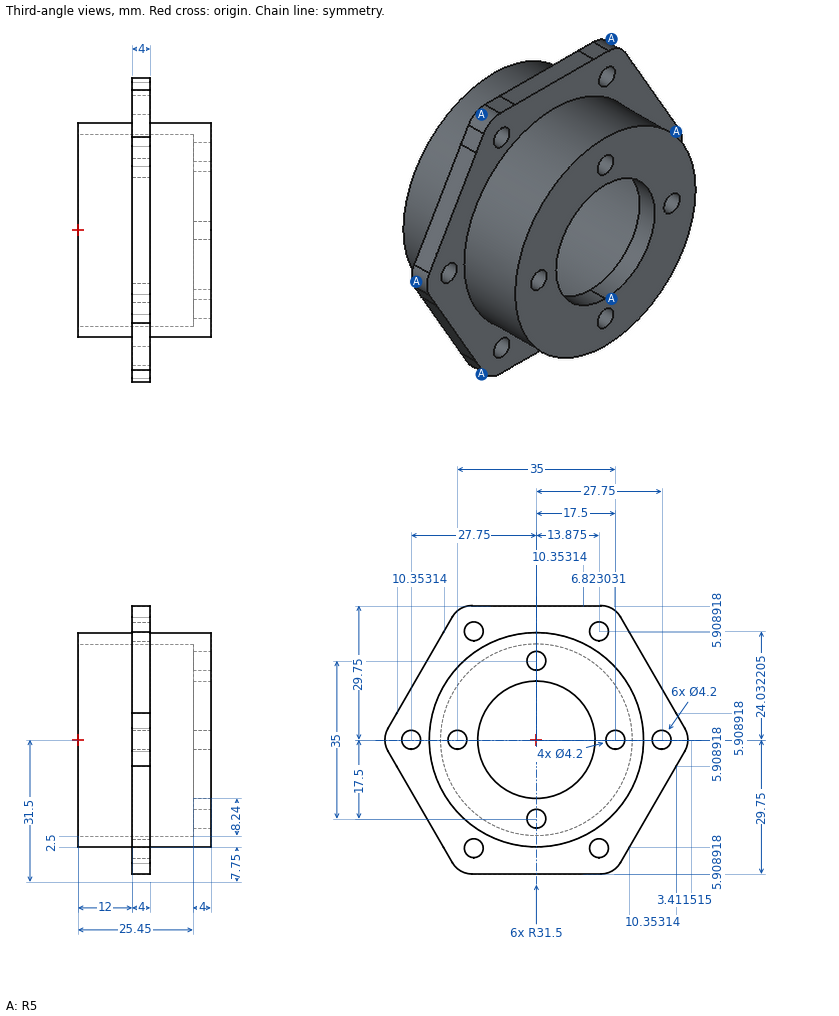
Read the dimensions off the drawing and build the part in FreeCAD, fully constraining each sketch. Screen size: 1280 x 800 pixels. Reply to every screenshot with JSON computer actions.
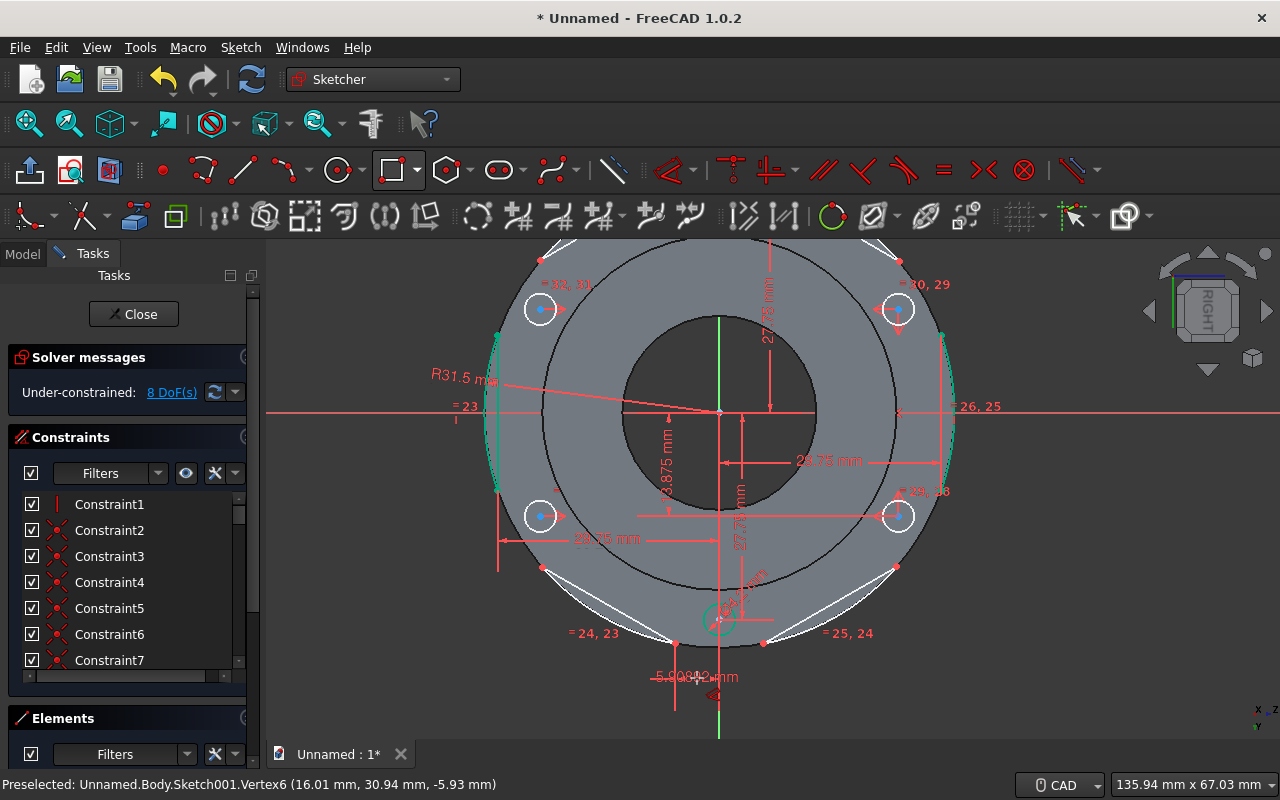
{"action": "left_click", "coordinate": [764, 644]}
{"action": "left_click", "coordinate": [742, 379]}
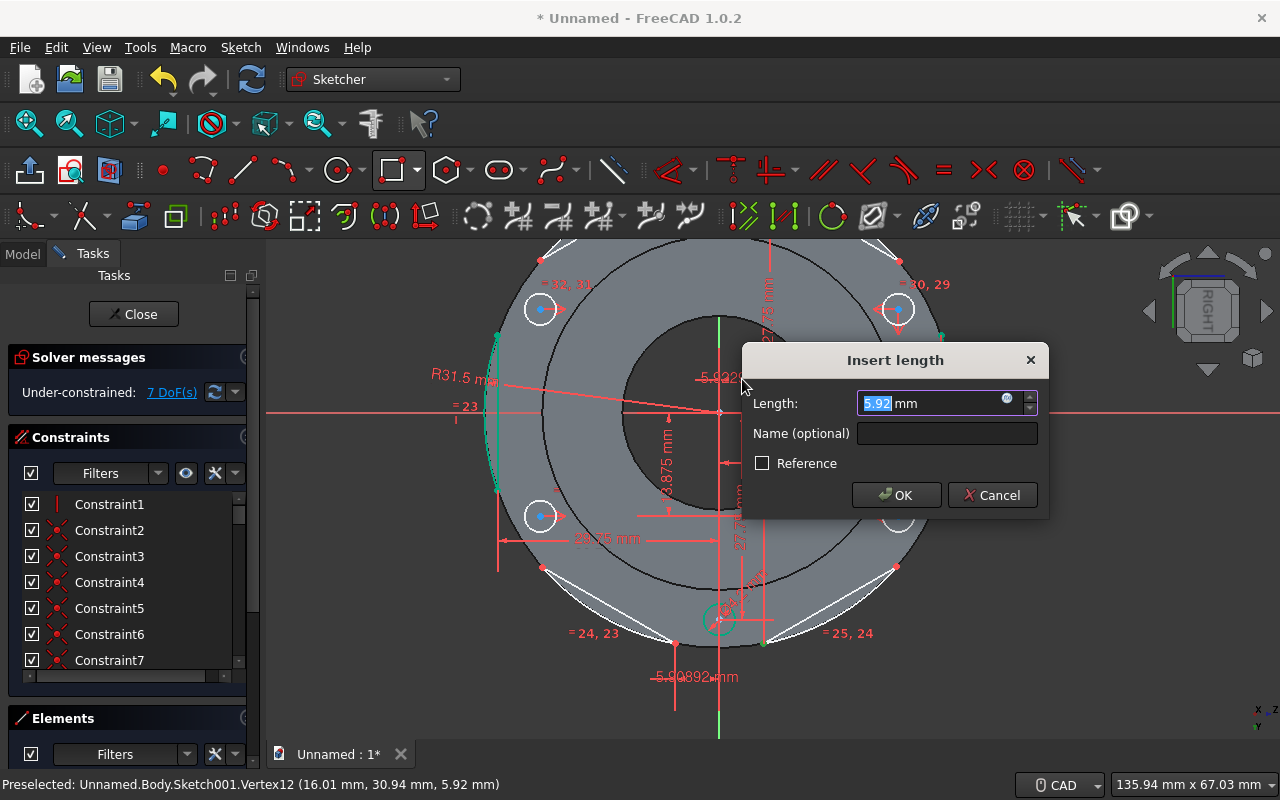
{"action": "type", "text": "5.908918"}
{"action": "key", "text": "Return"}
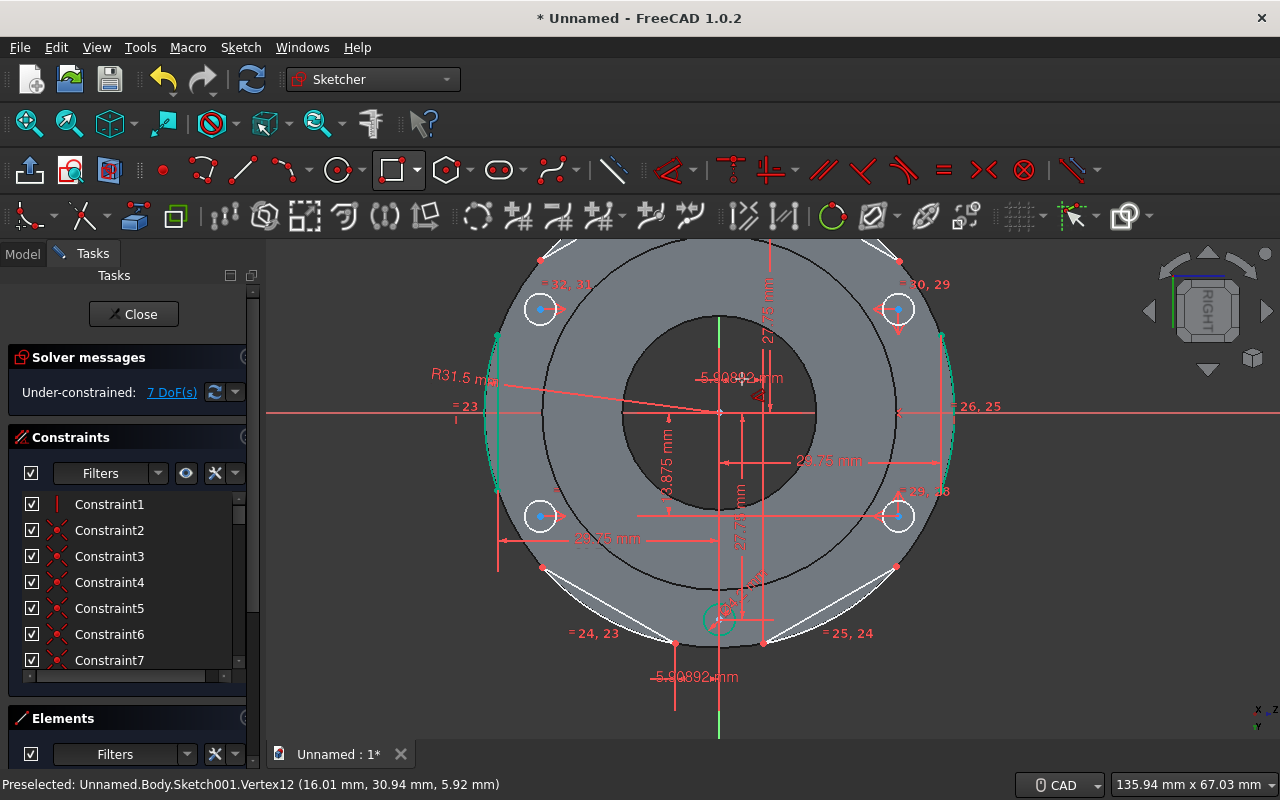
{"action": "scroll", "coordinate": [674, 644], "scroll_direction": "down", "scroll_amount": 2}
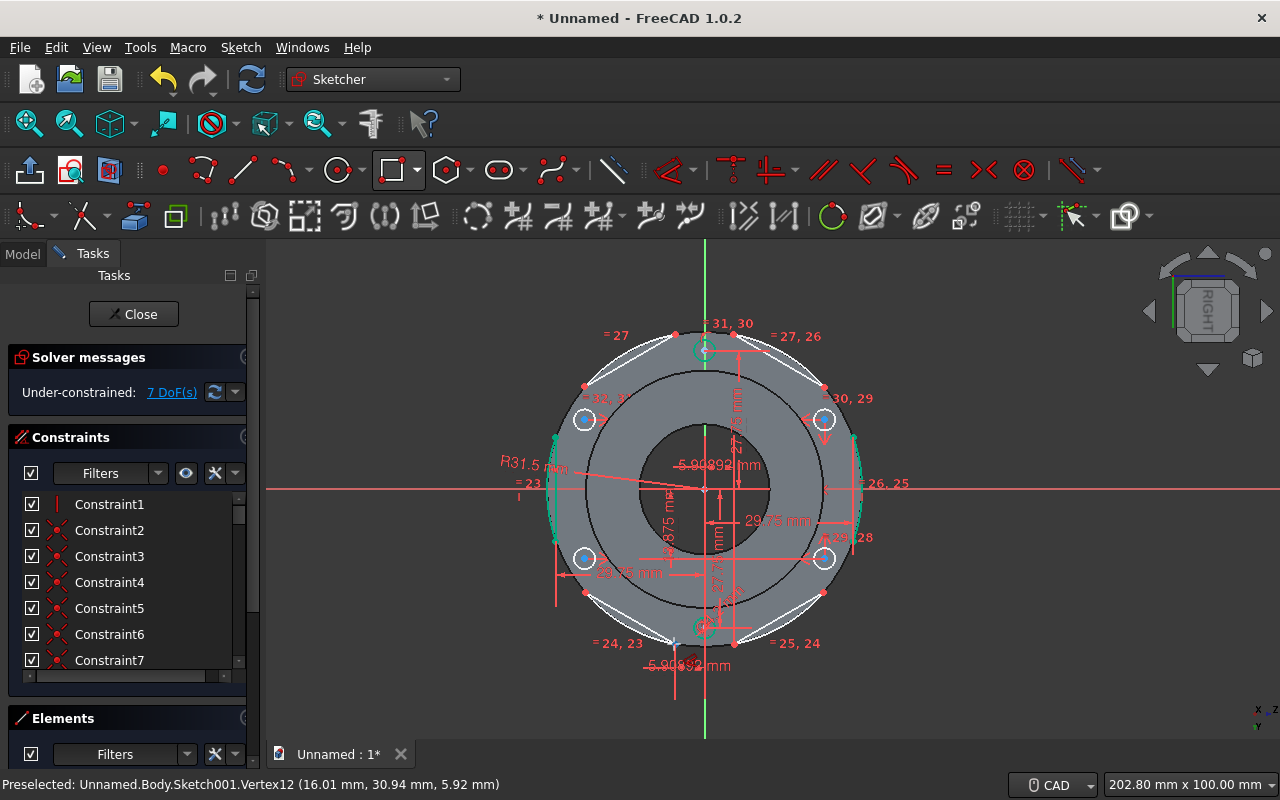
{"action": "scroll", "coordinate": [734, 335], "scroll_direction": "up", "scroll_amount": 2}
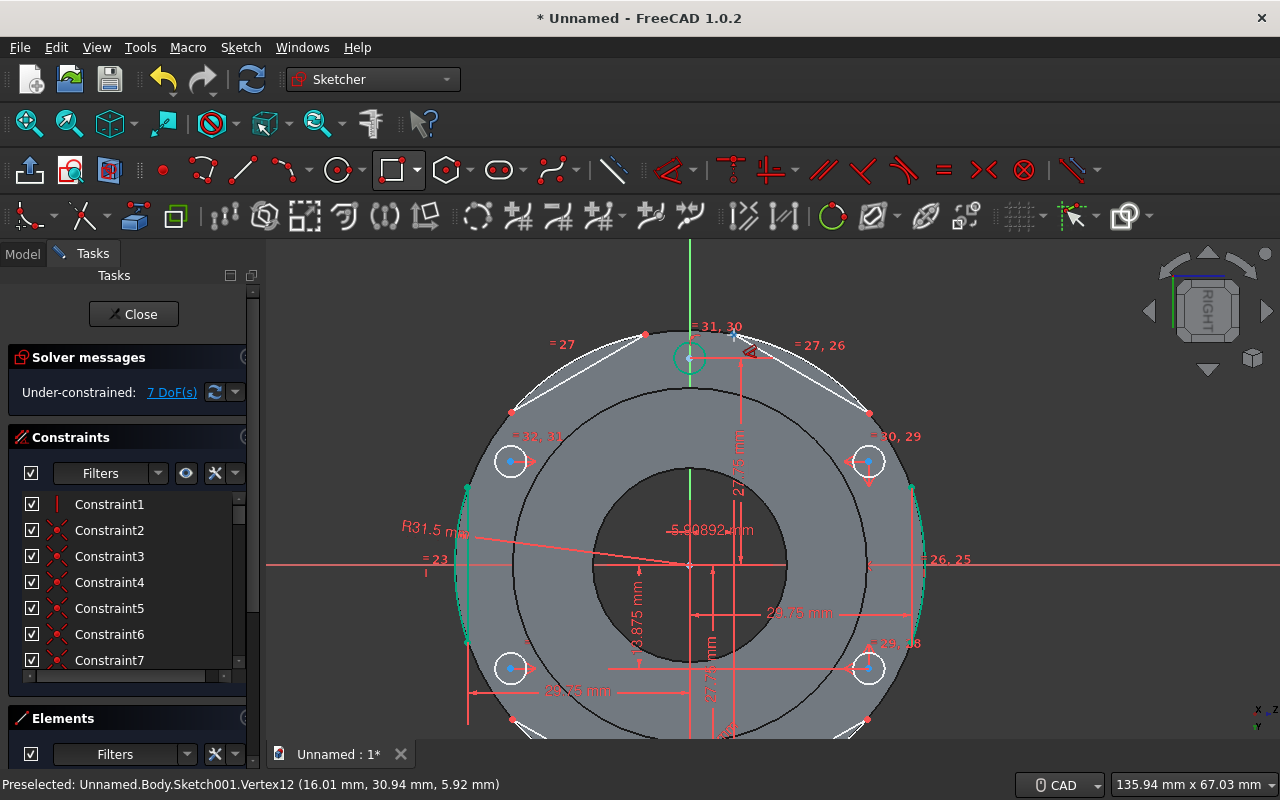
{"action": "left_click", "coordinate": [734, 334]}
{"action": "left_click", "coordinate": [712, 300]}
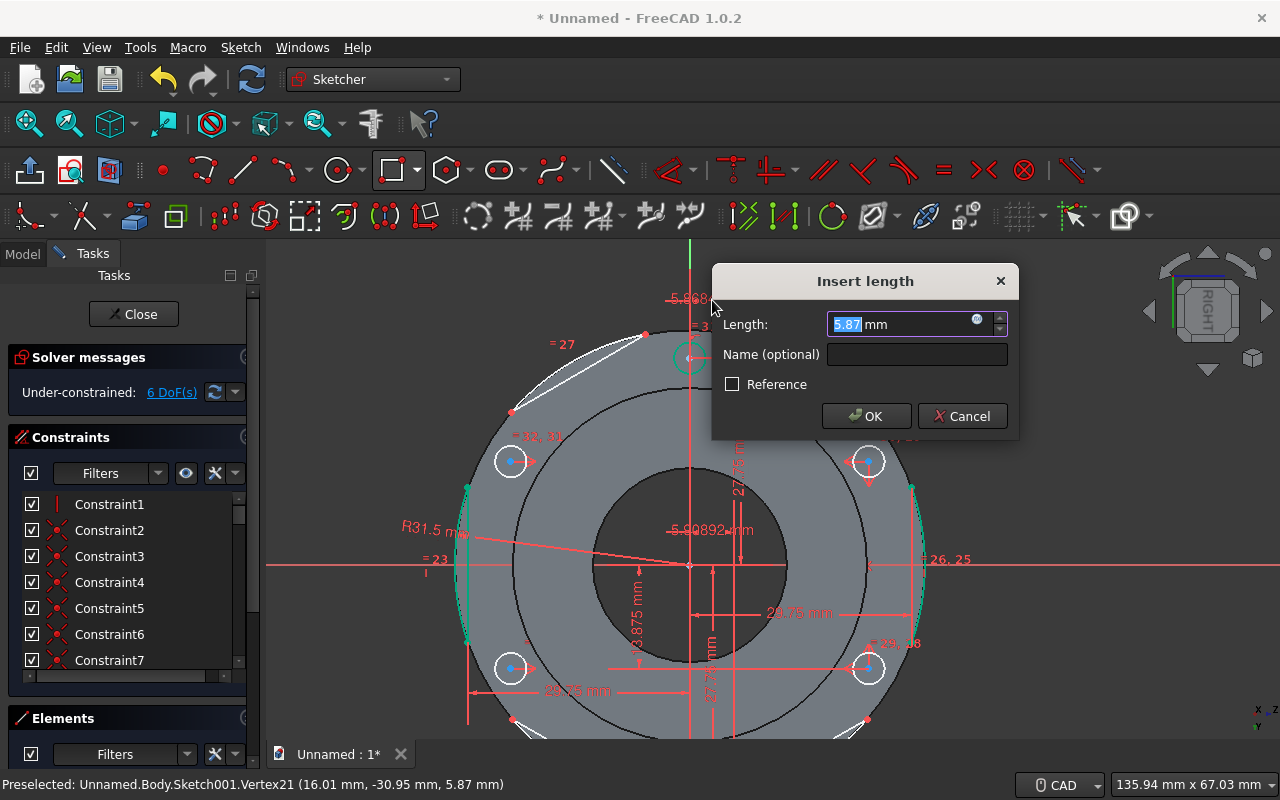
{"action": "type", "text": "5.908918"}
{"action": "key", "text": "Return"}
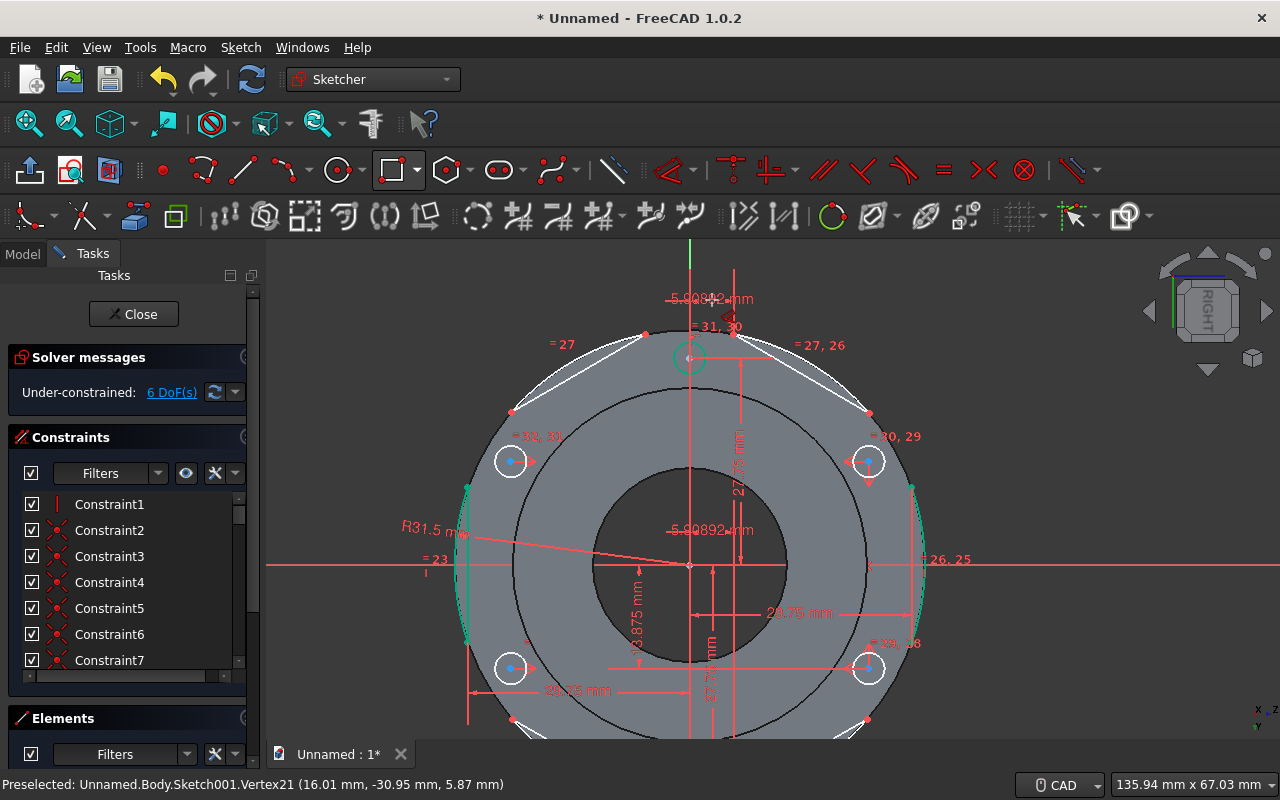
{"action": "left_click", "coordinate": [646, 334]}
{"action": "left_click", "coordinate": [668, 276]}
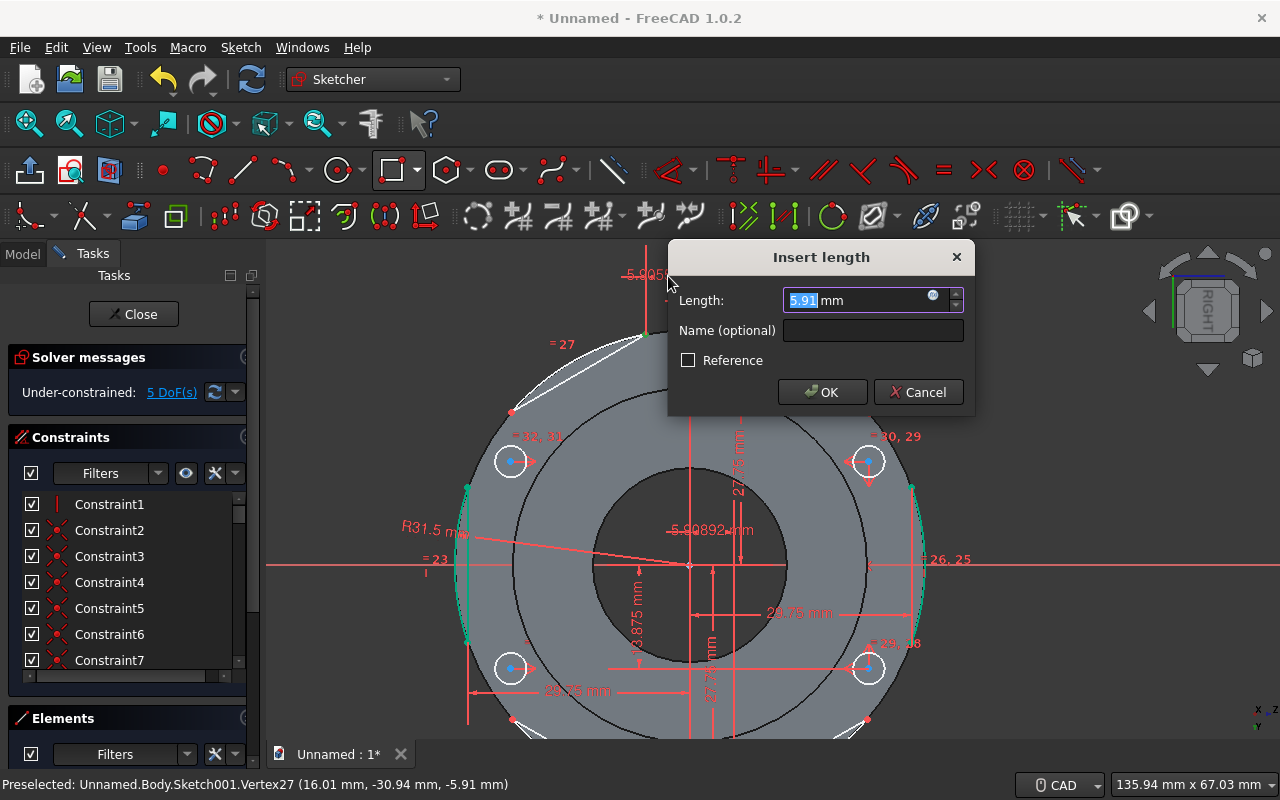
{"action": "type", "text": "5.908918"}
{"action": "key", "text": "Return"}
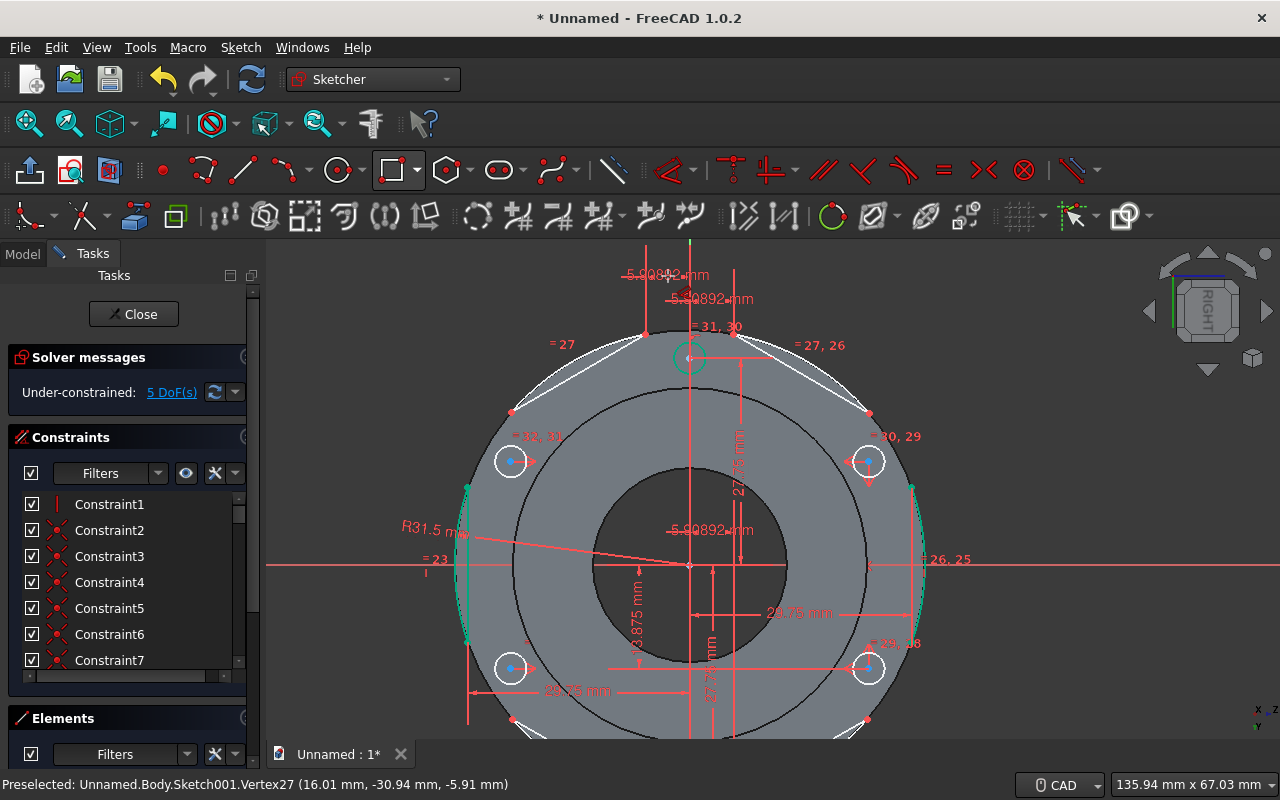
{"action": "scroll", "coordinate": [734, 334], "scroll_direction": "down", "scroll_amount": 2}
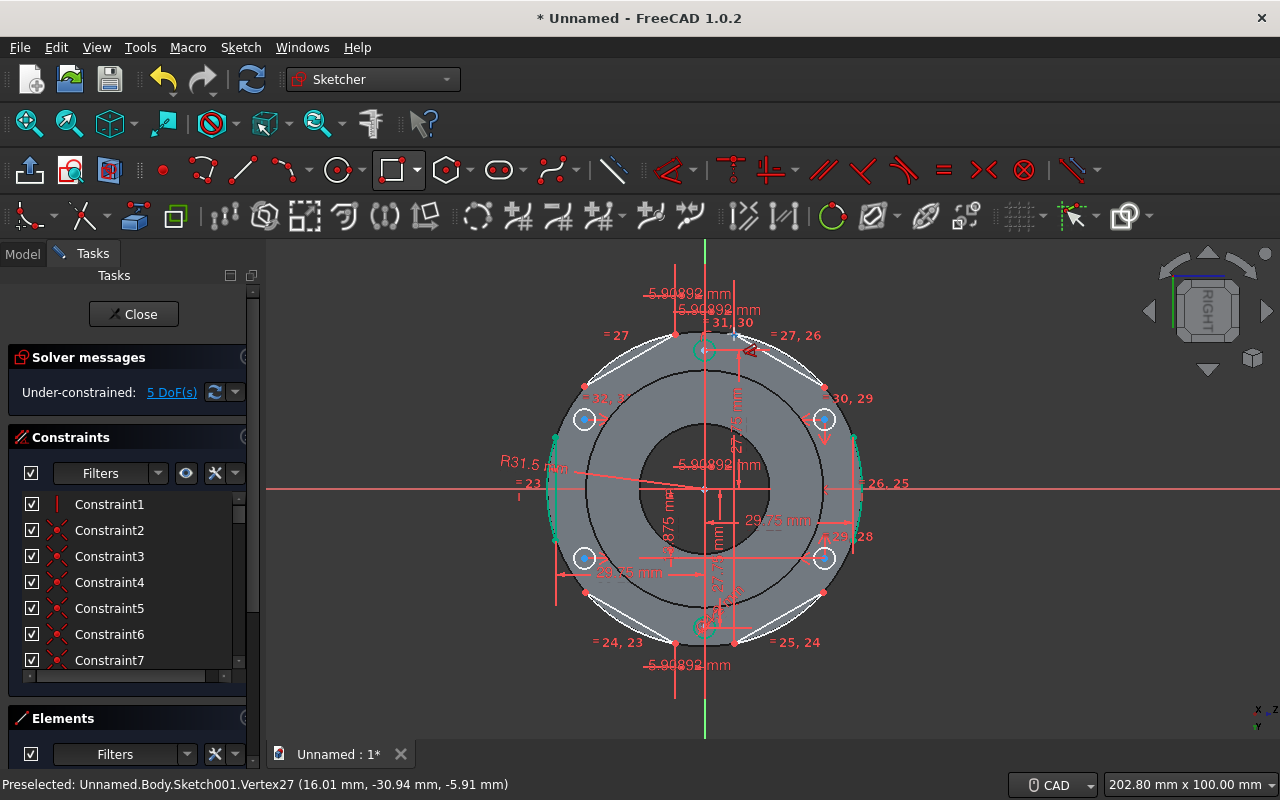
{"action": "scroll", "coordinate": [648, 628], "scroll_direction": "up", "scroll_amount": 4}